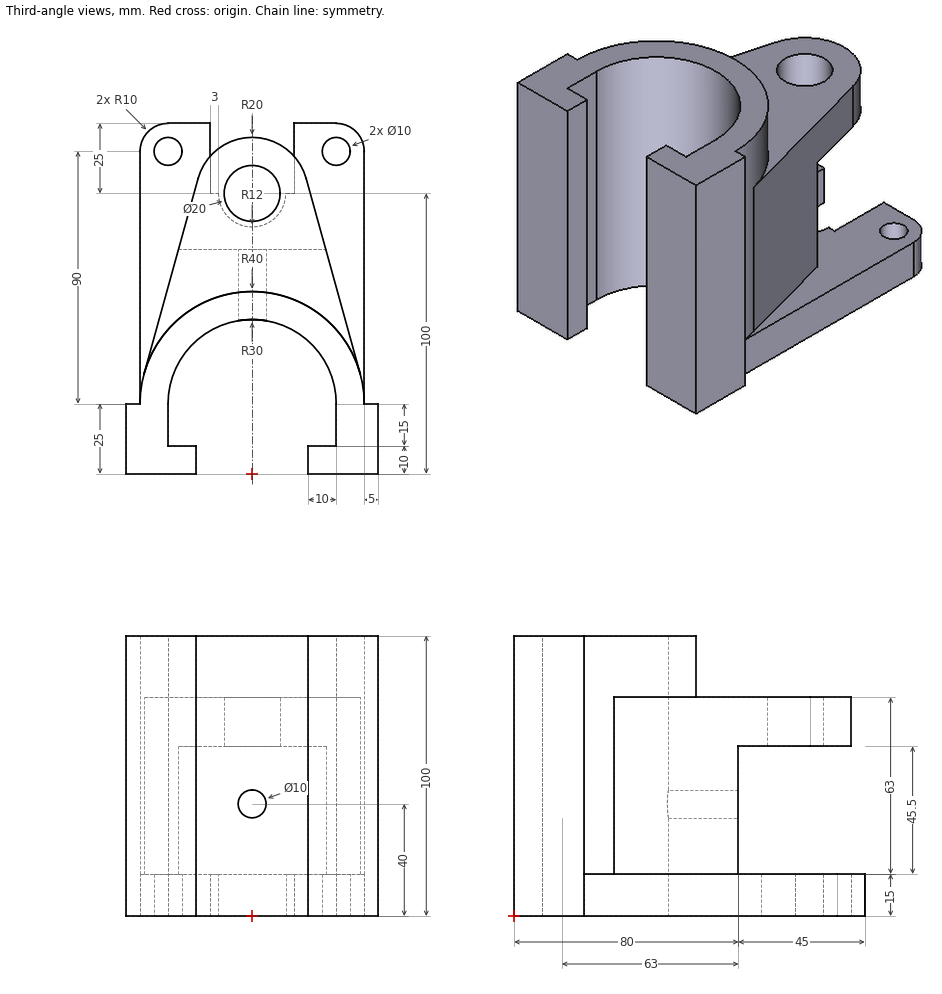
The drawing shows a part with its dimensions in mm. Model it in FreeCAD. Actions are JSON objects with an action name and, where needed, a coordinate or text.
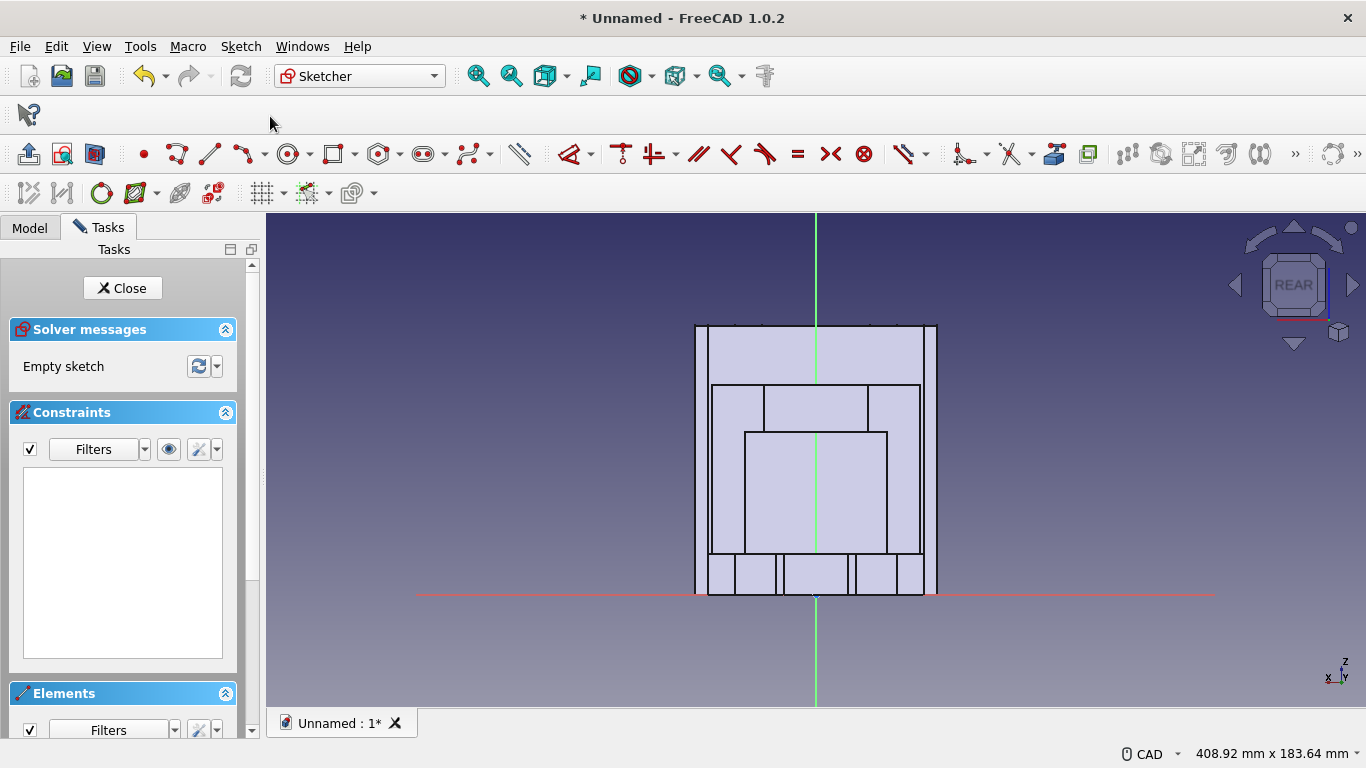
{"action": "key", "text": "q s"}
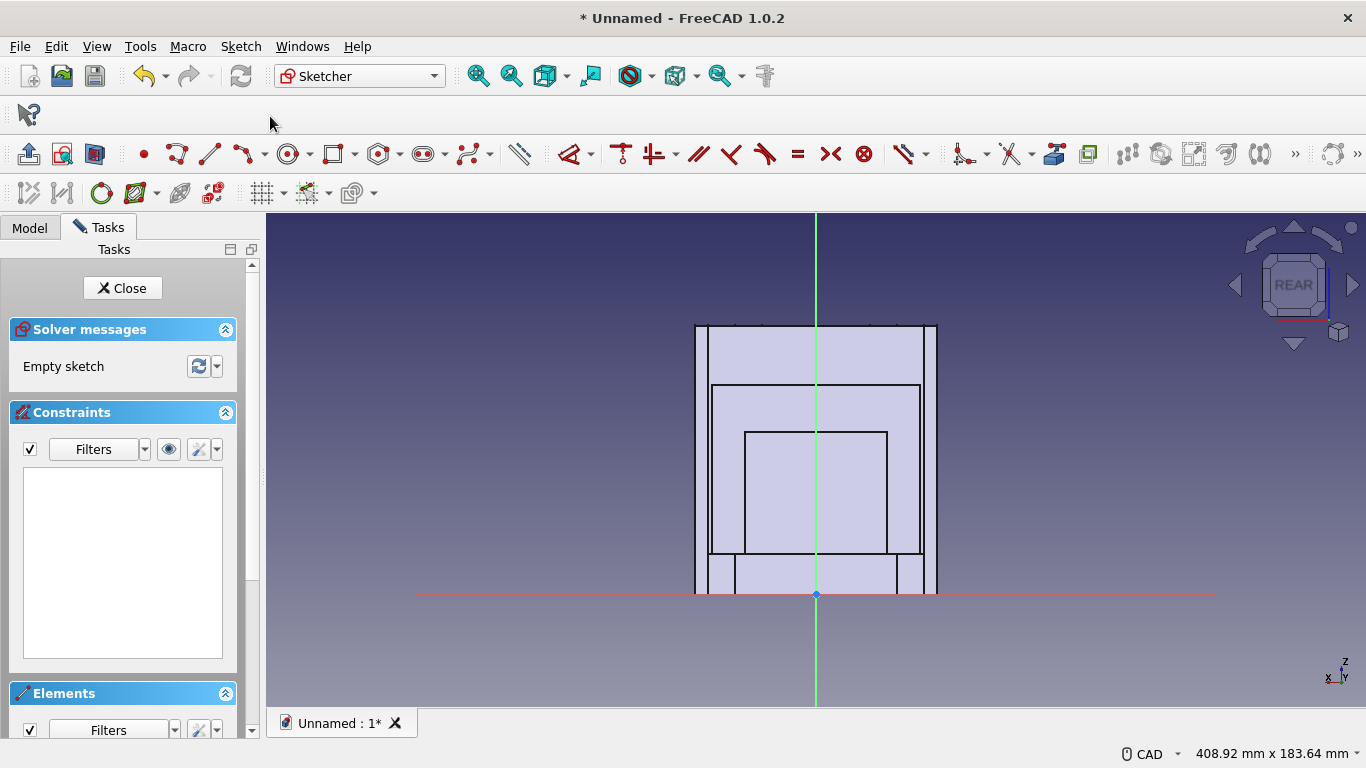
{"action": "scroll", "coordinate": [823, 490], "scroll_direction": "up", "scroll_amount": 12}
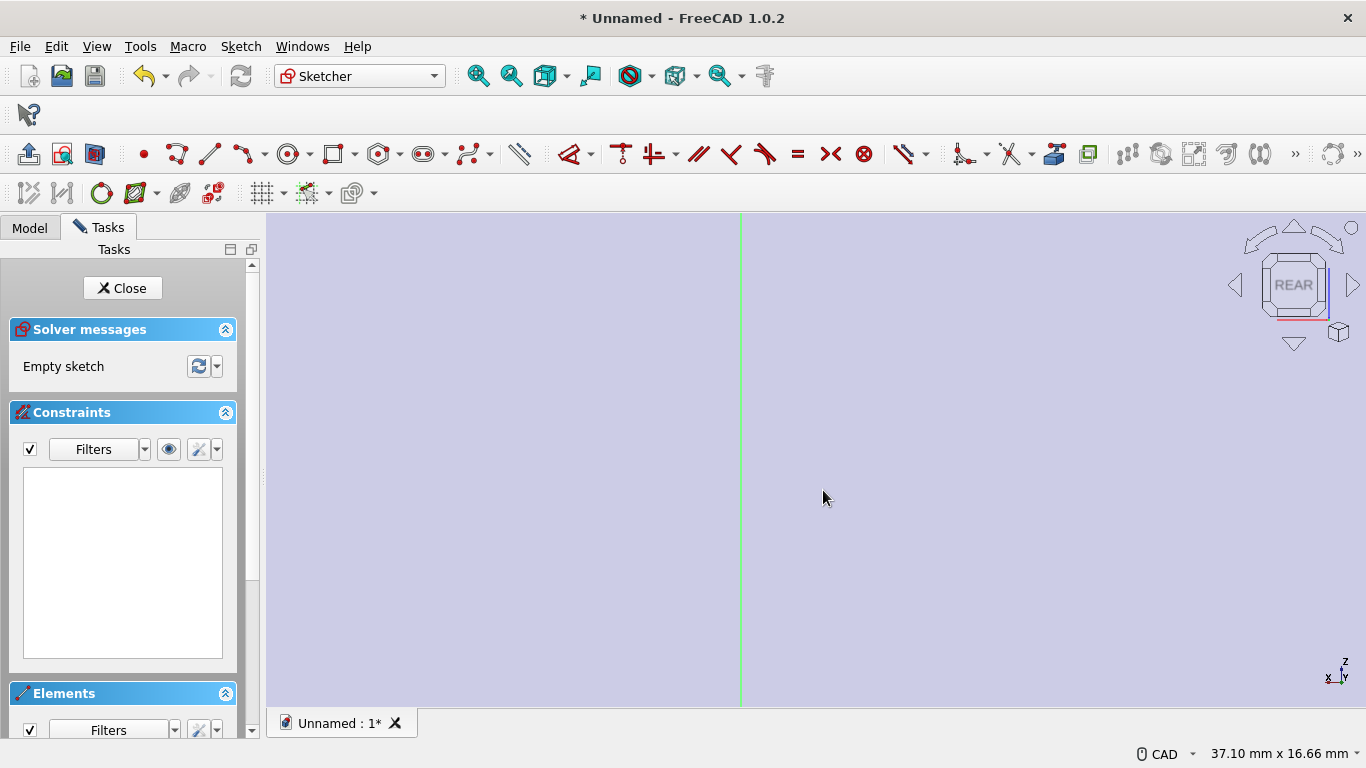
{"action": "key", "text": "g c"}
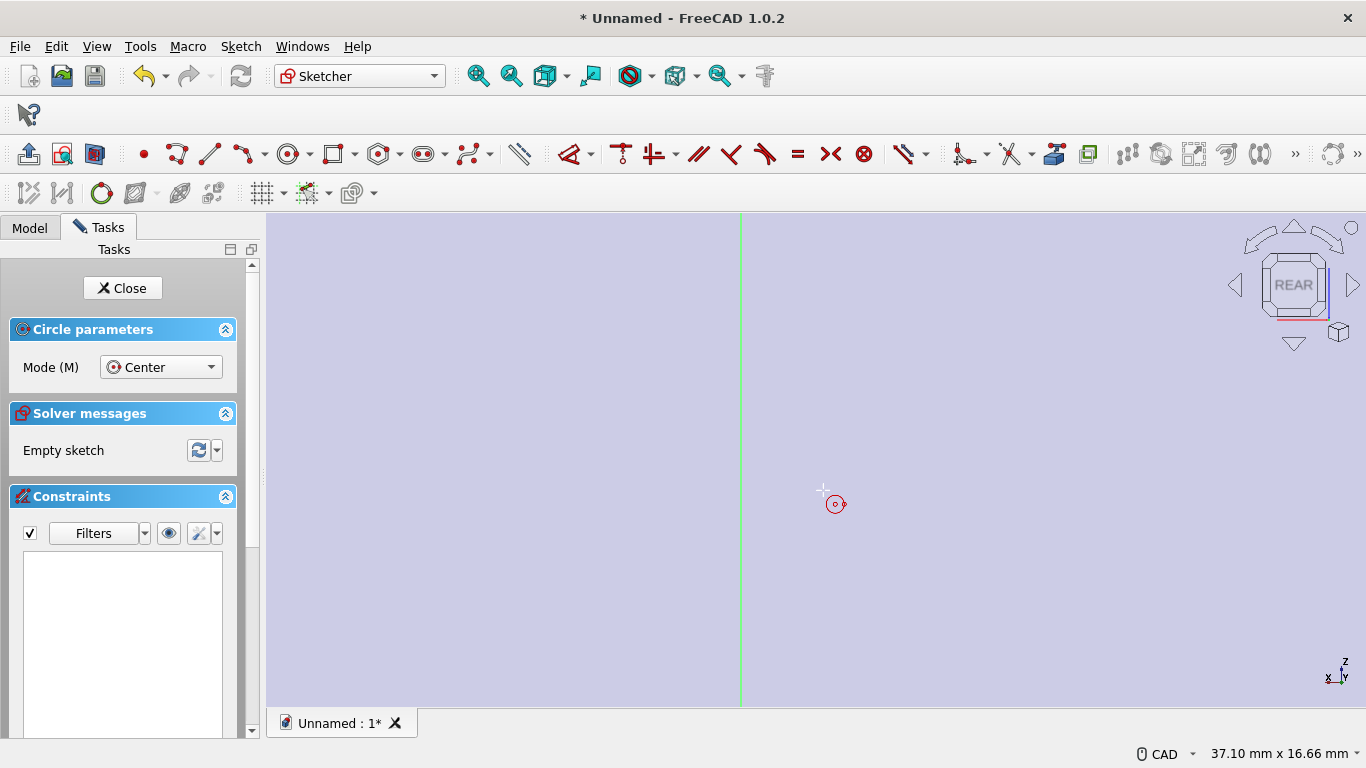
{"action": "left_click", "coordinate": [741, 450]}
{"action": "mouse_move", "coordinate": [846, 345]}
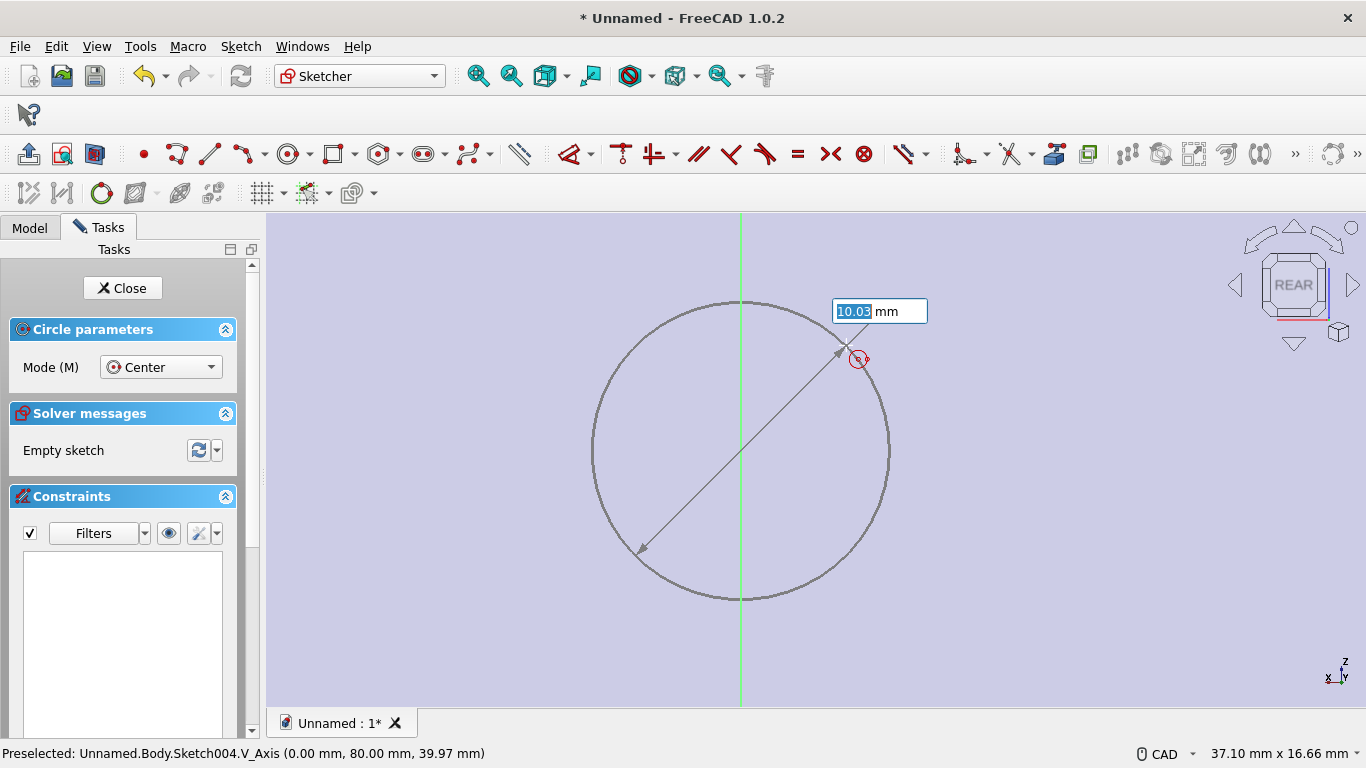
{"action": "type", "text": "10"}
{"action": "key", "text": "Return"}
{"action": "key", "text": "Escape"}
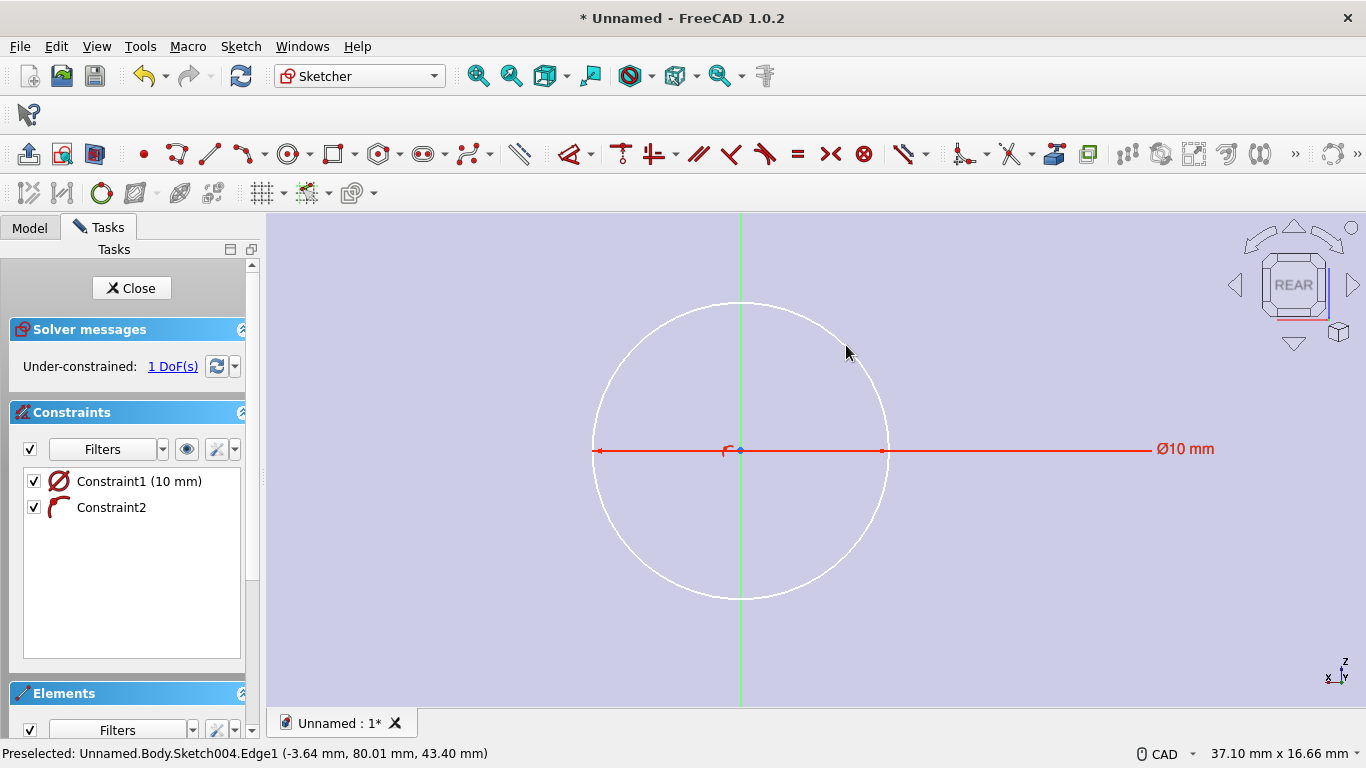
{"action": "left_click", "coordinate": [568, 154]}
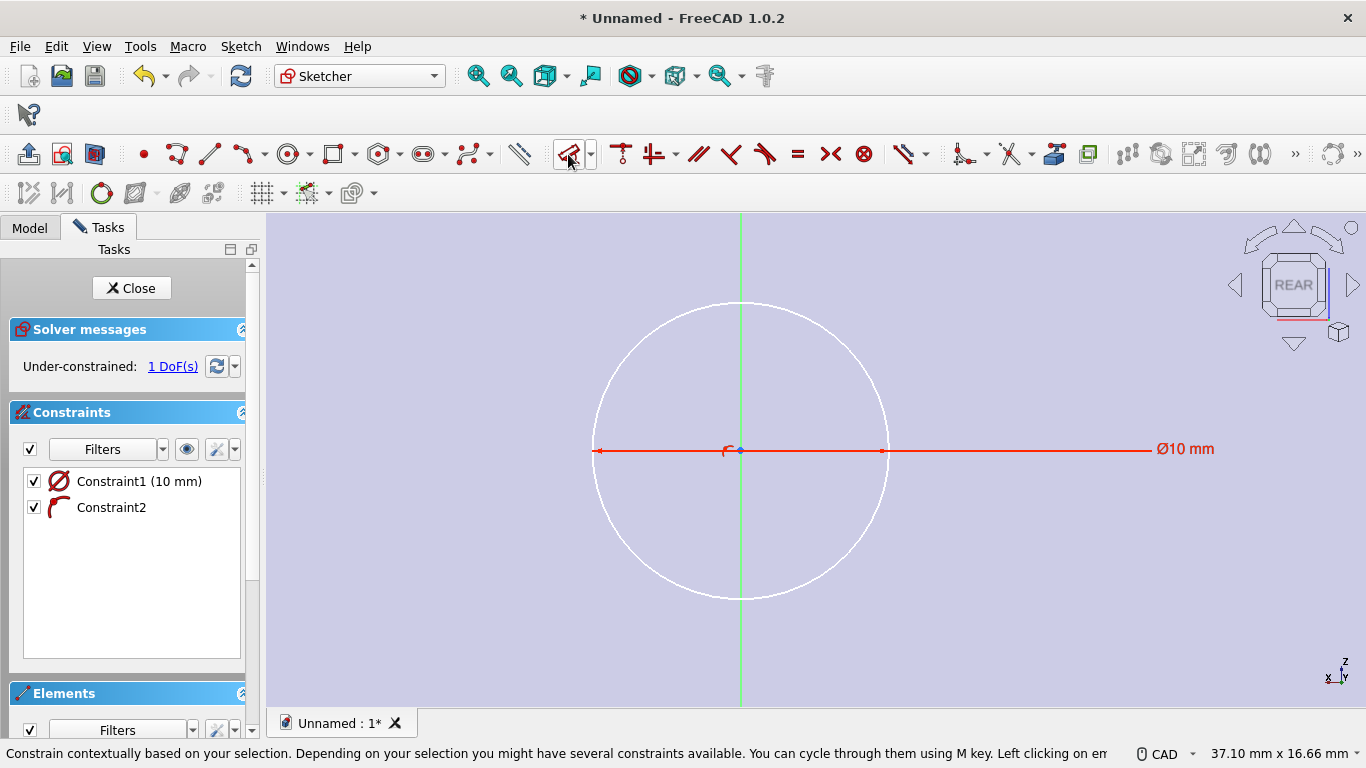
{"action": "left_click", "coordinate": [741, 451]}
{"action": "left_click", "coordinate": [775, 565]}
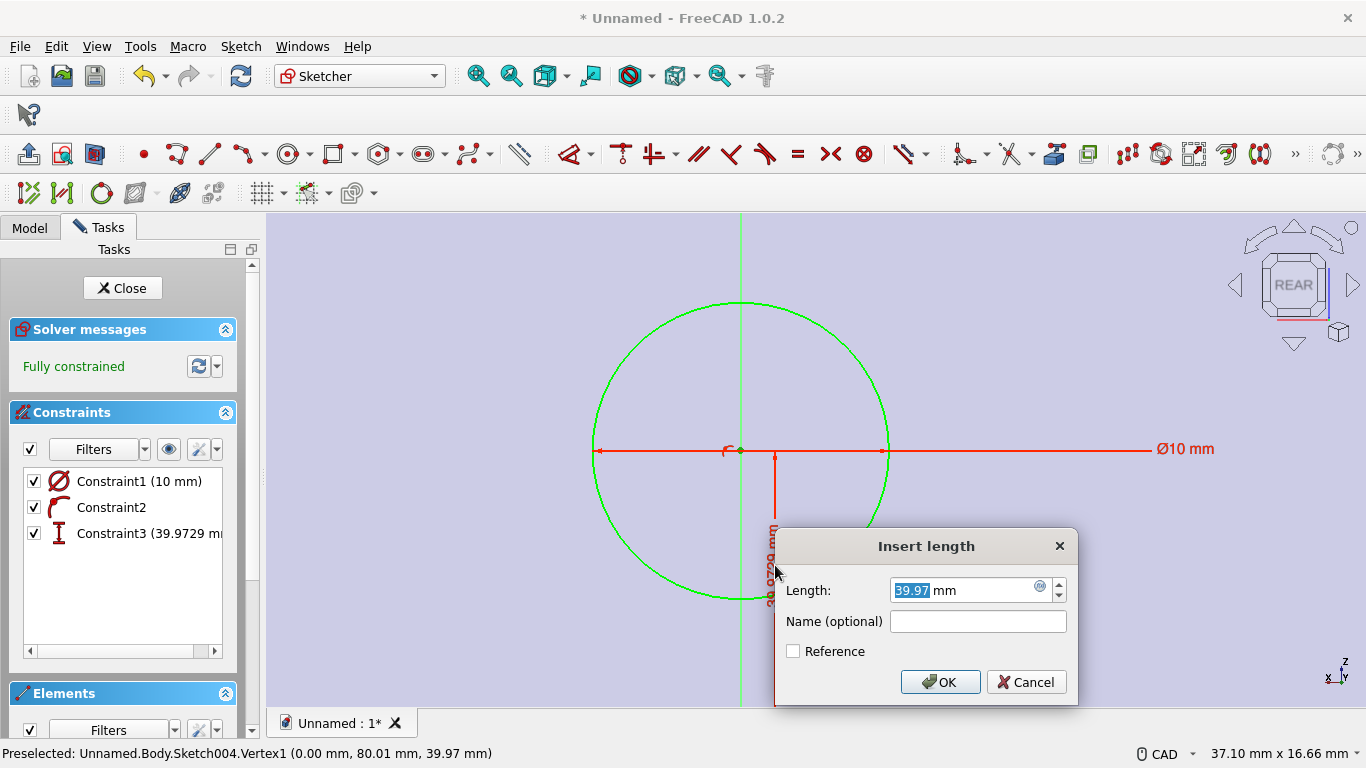
{"action": "type", "text": "40"}
{"action": "key", "text": "Return"}
{"action": "key", "text": "Escape"}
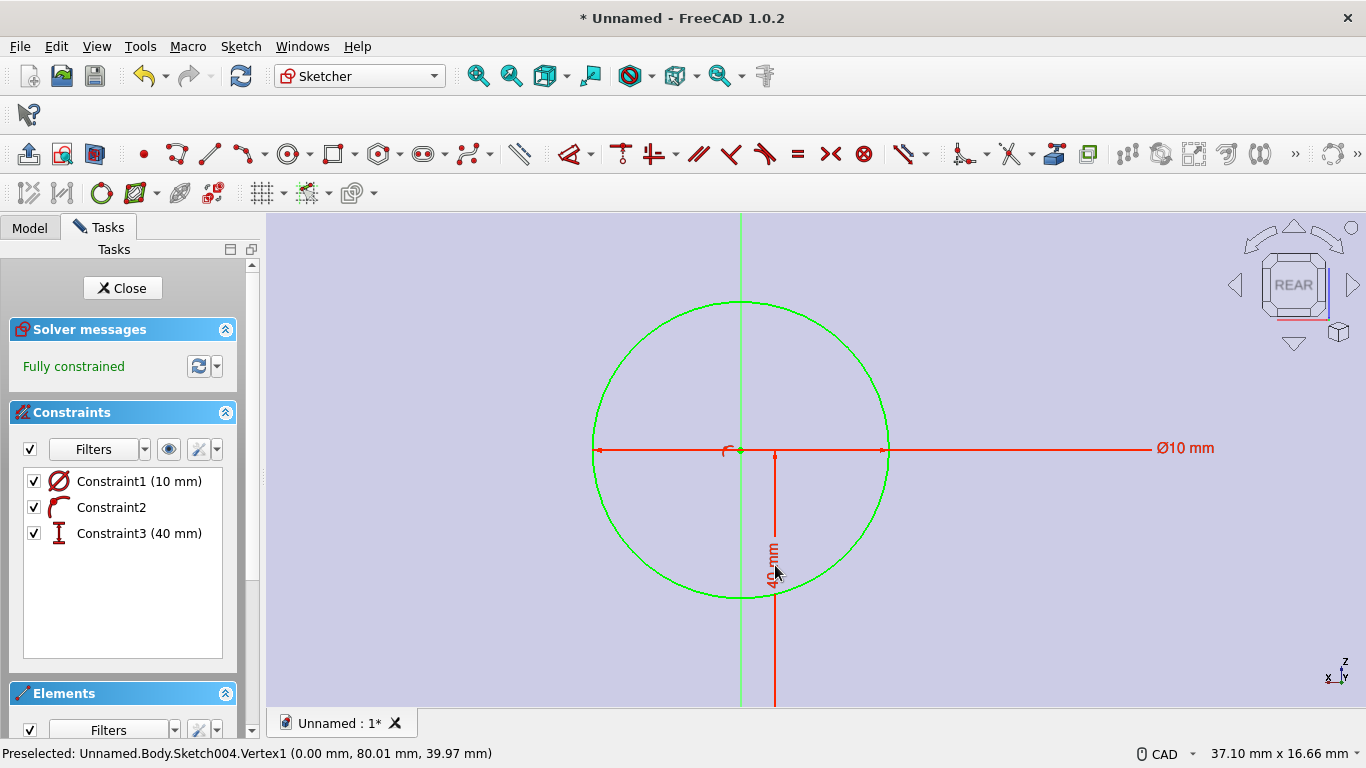
{"action": "left_click", "coordinate": [123, 288]}